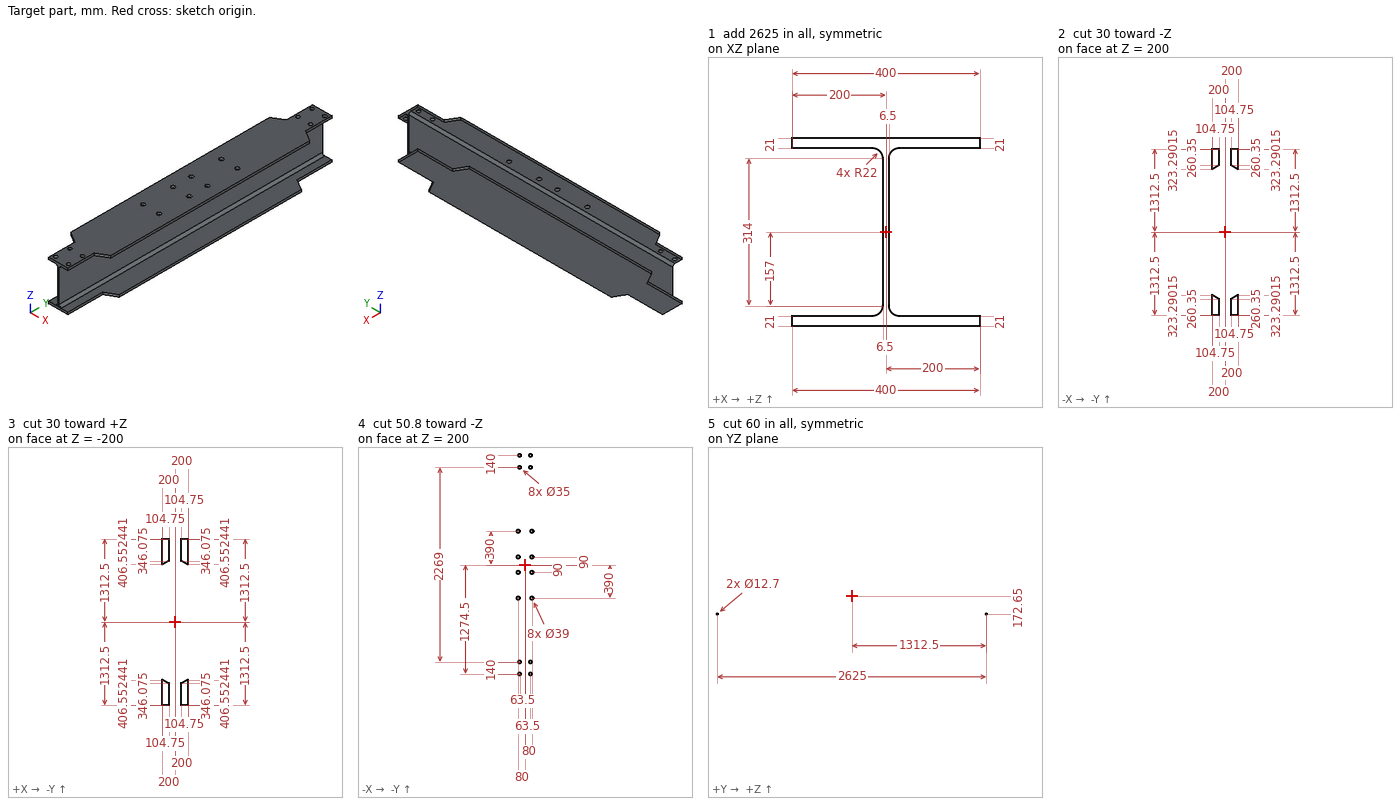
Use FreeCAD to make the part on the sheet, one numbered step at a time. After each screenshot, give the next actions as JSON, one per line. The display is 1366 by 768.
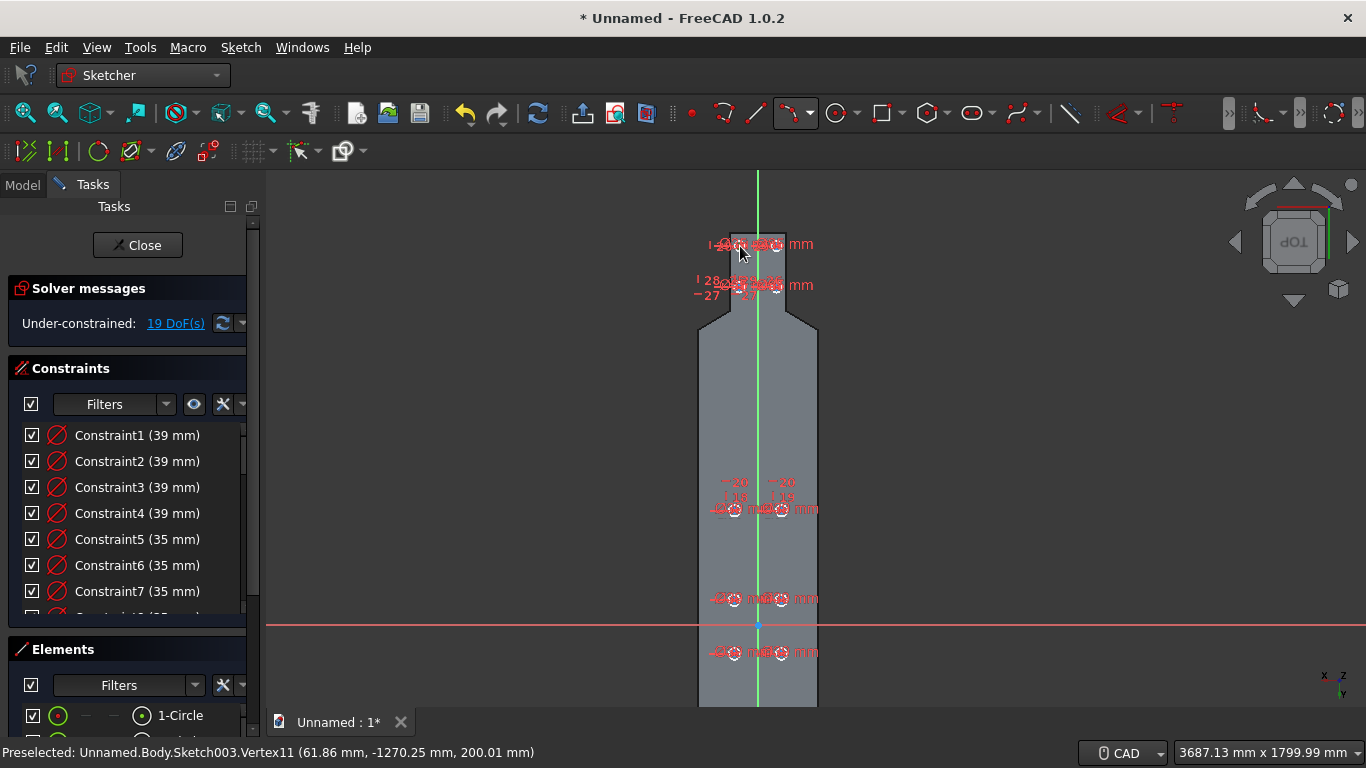
{"action": "left_click", "coordinate": [777, 246]}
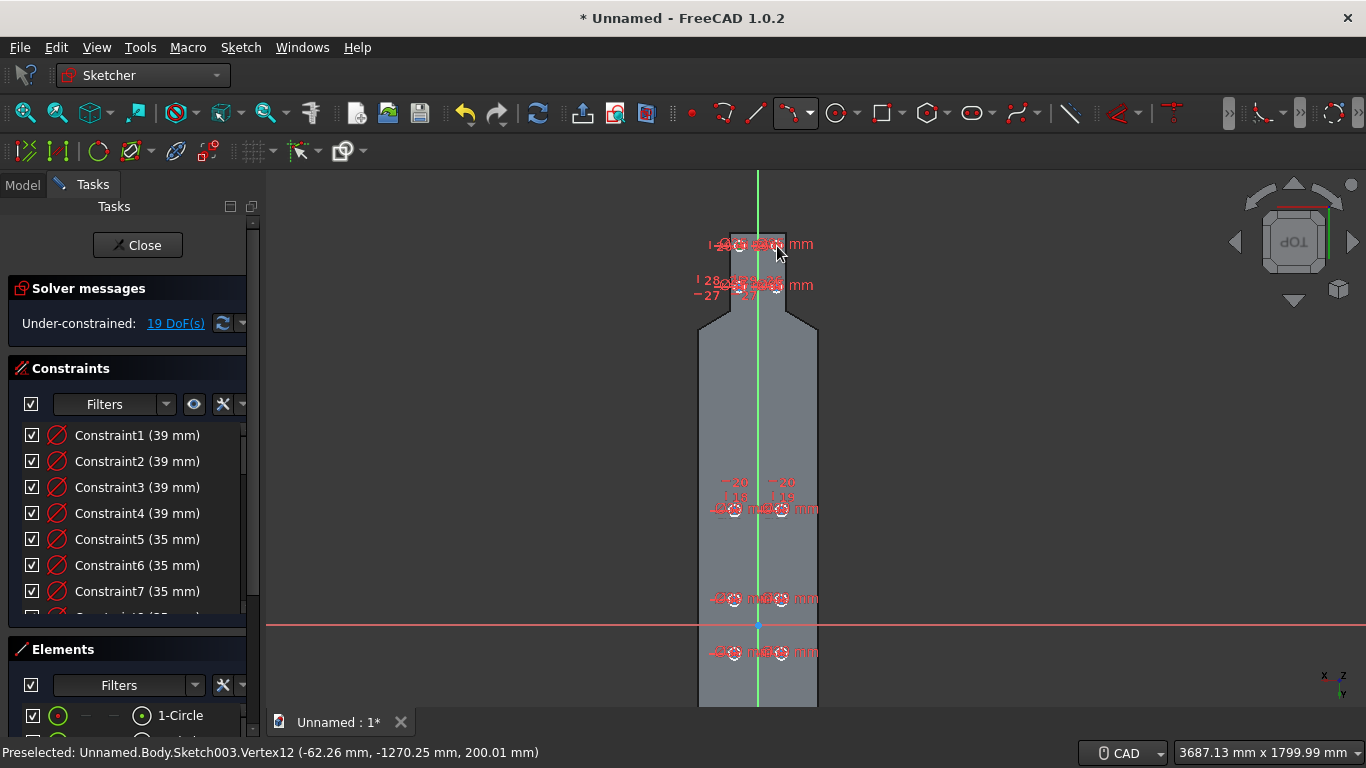
{"action": "key", "text": "h"}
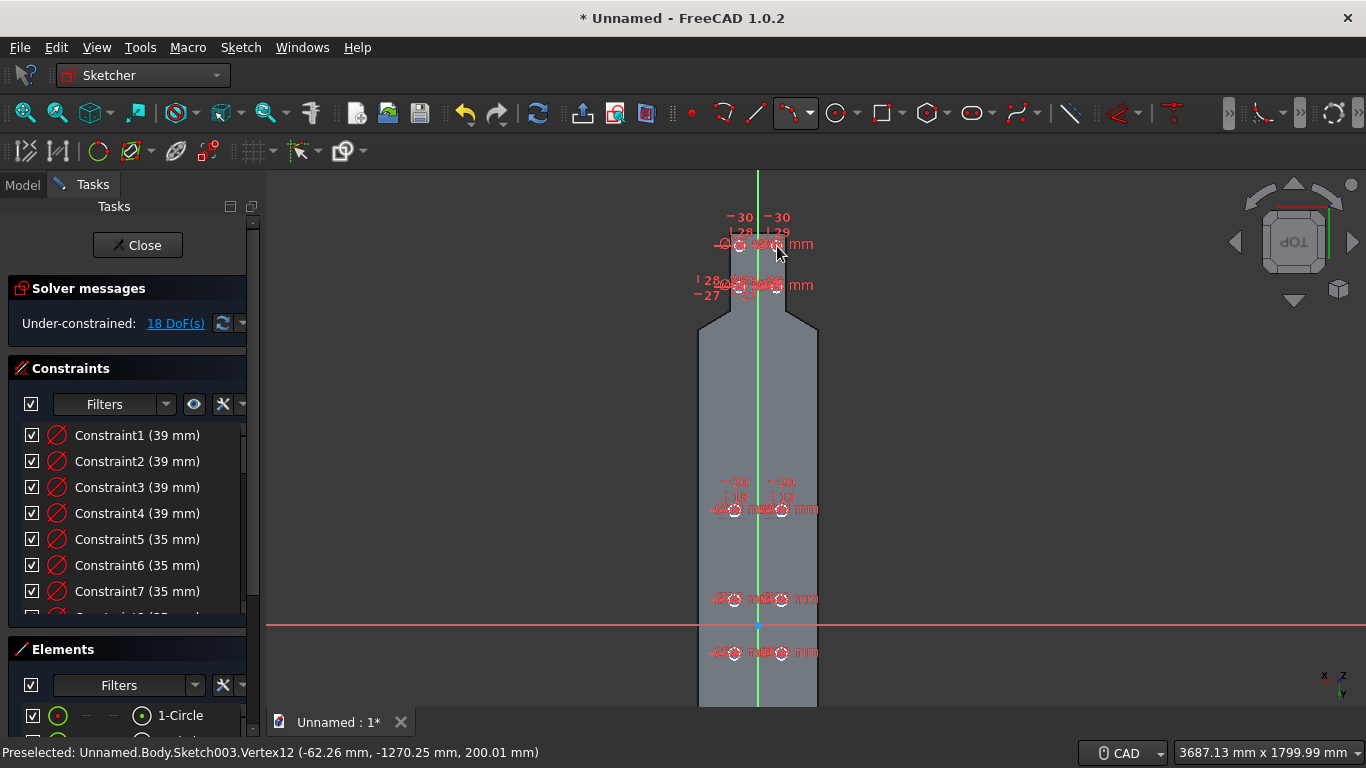
{"action": "scroll", "coordinate": [739, 286], "scroll_direction": "down", "scroll_amount": 4}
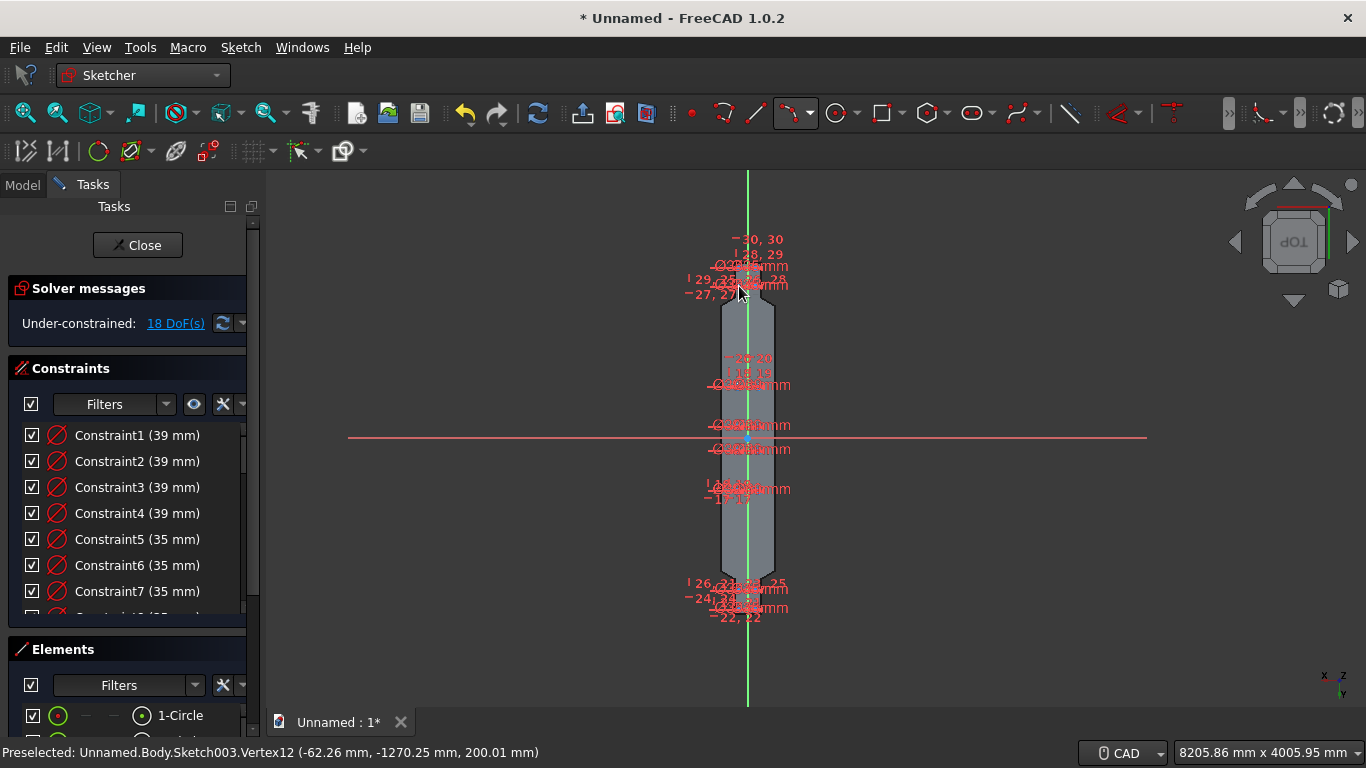
{"action": "left_click", "coordinate": [758, 491]}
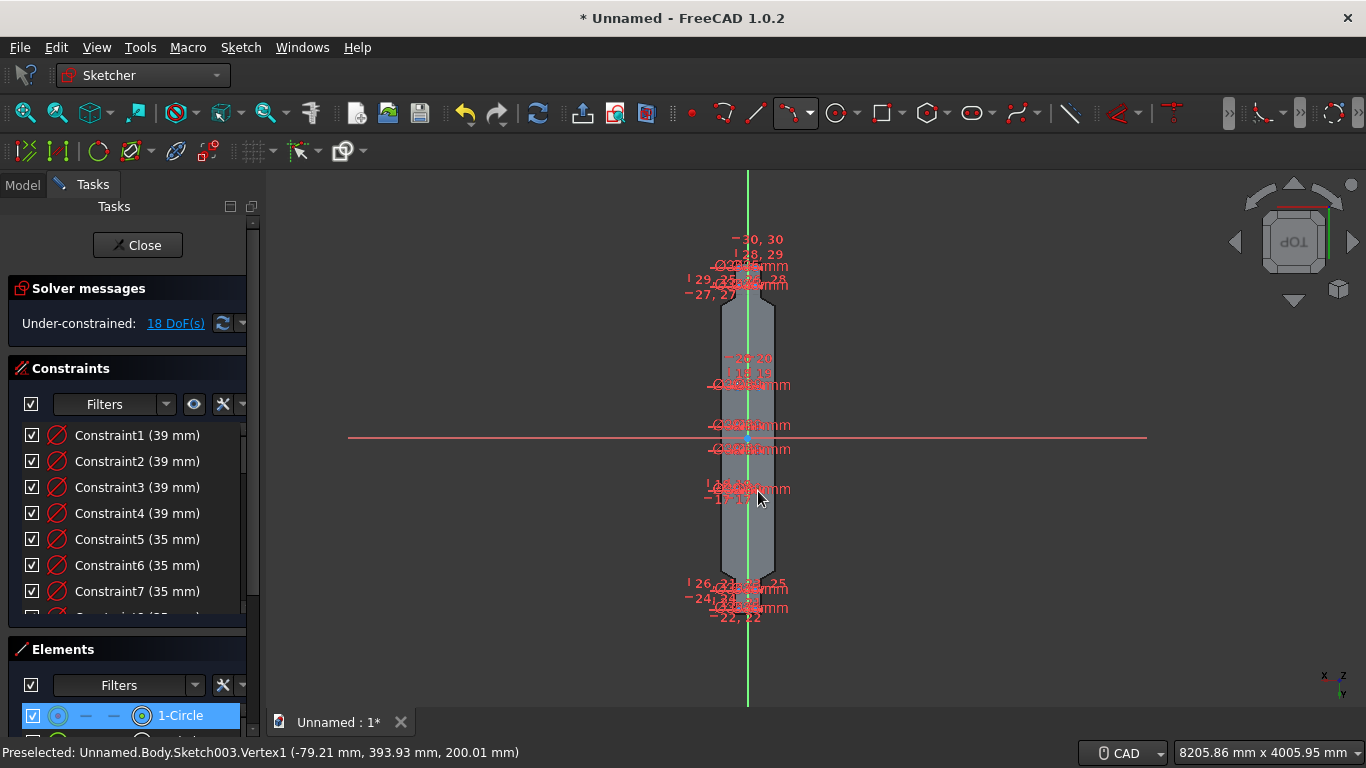
{"action": "left_click", "coordinate": [758, 451]}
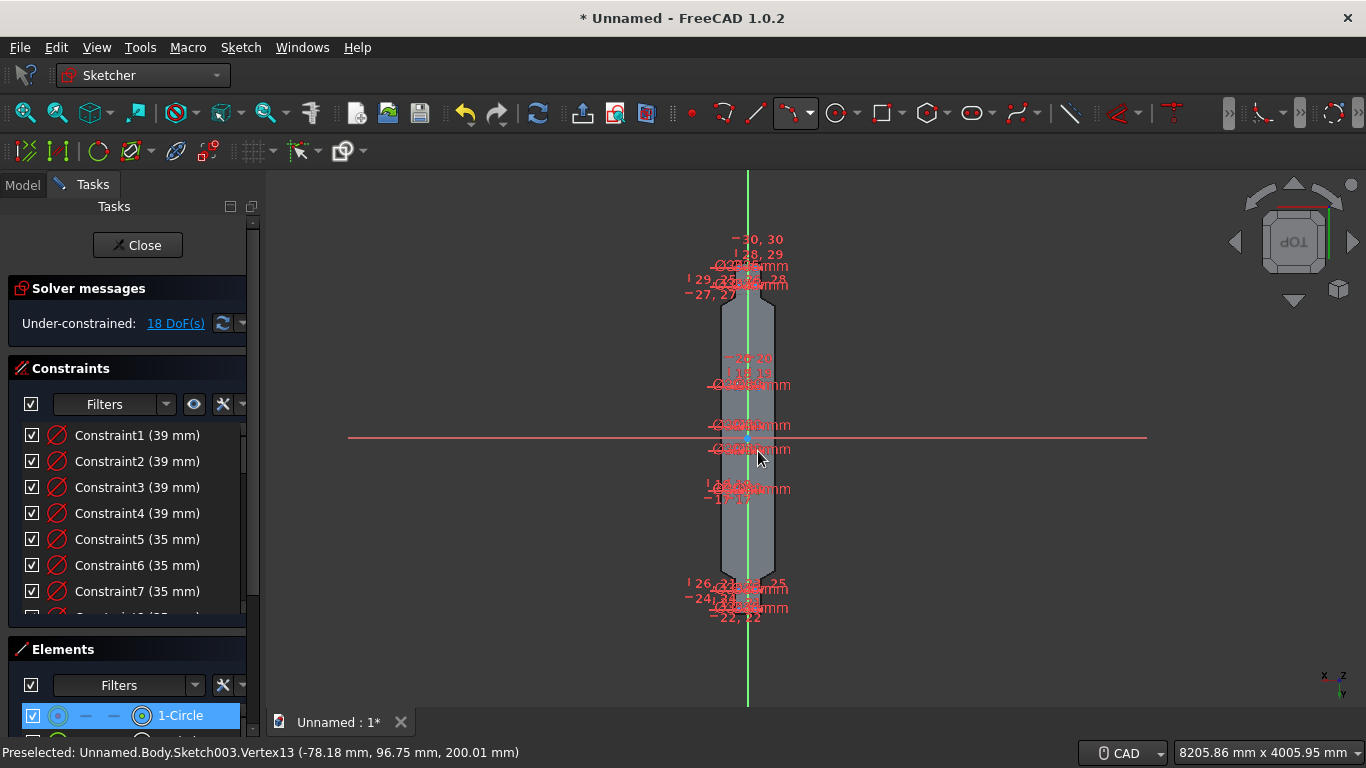
{"action": "key", "text": "v"}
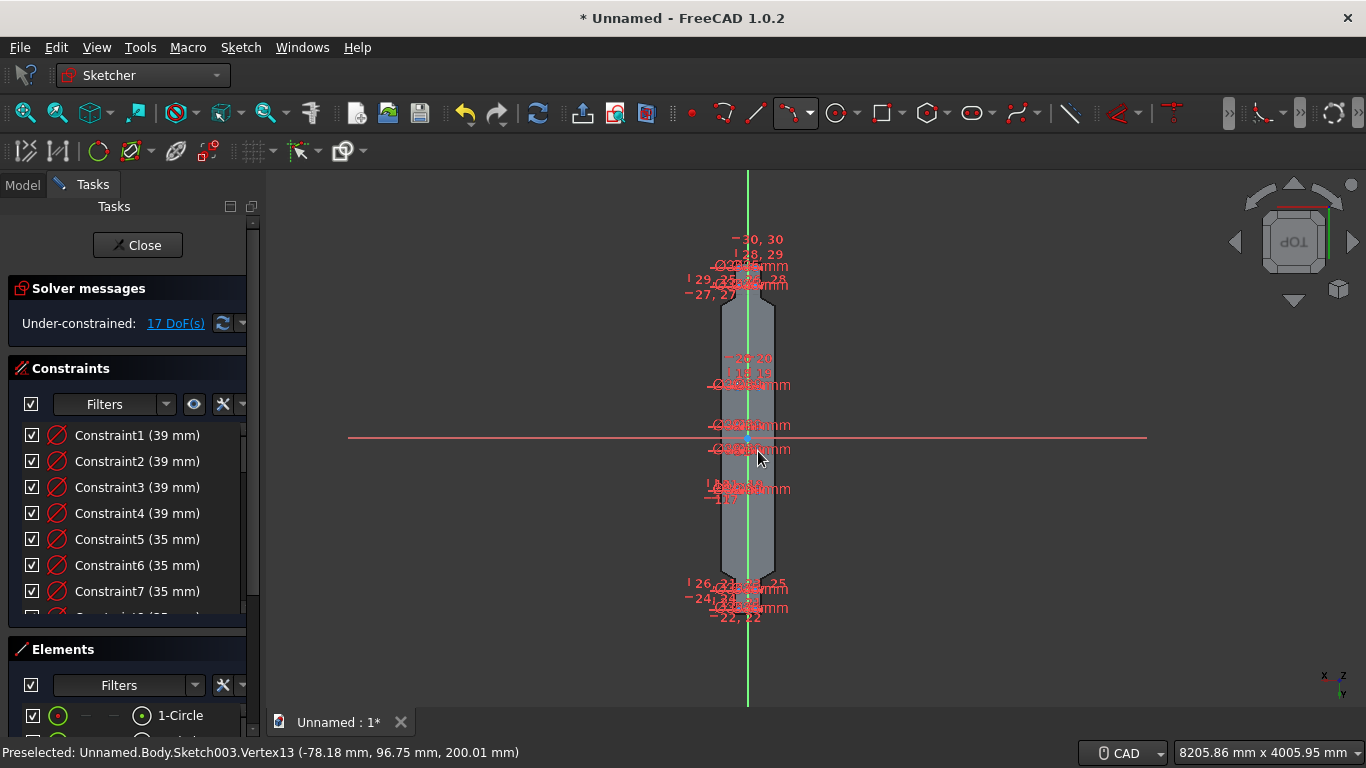
{"action": "left_click", "coordinate": [737, 491]}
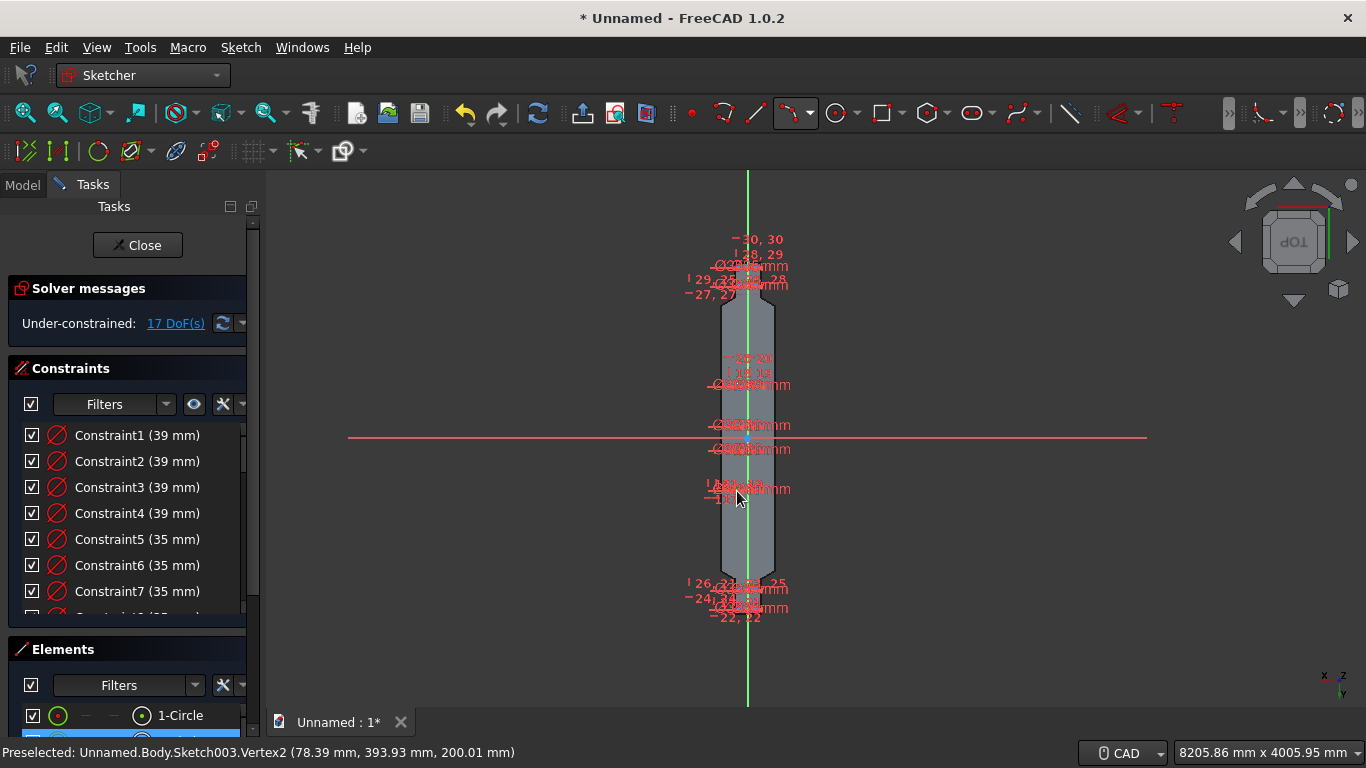
{"action": "scroll", "coordinate": [737, 451], "scroll_direction": "up", "scroll_amount": 4}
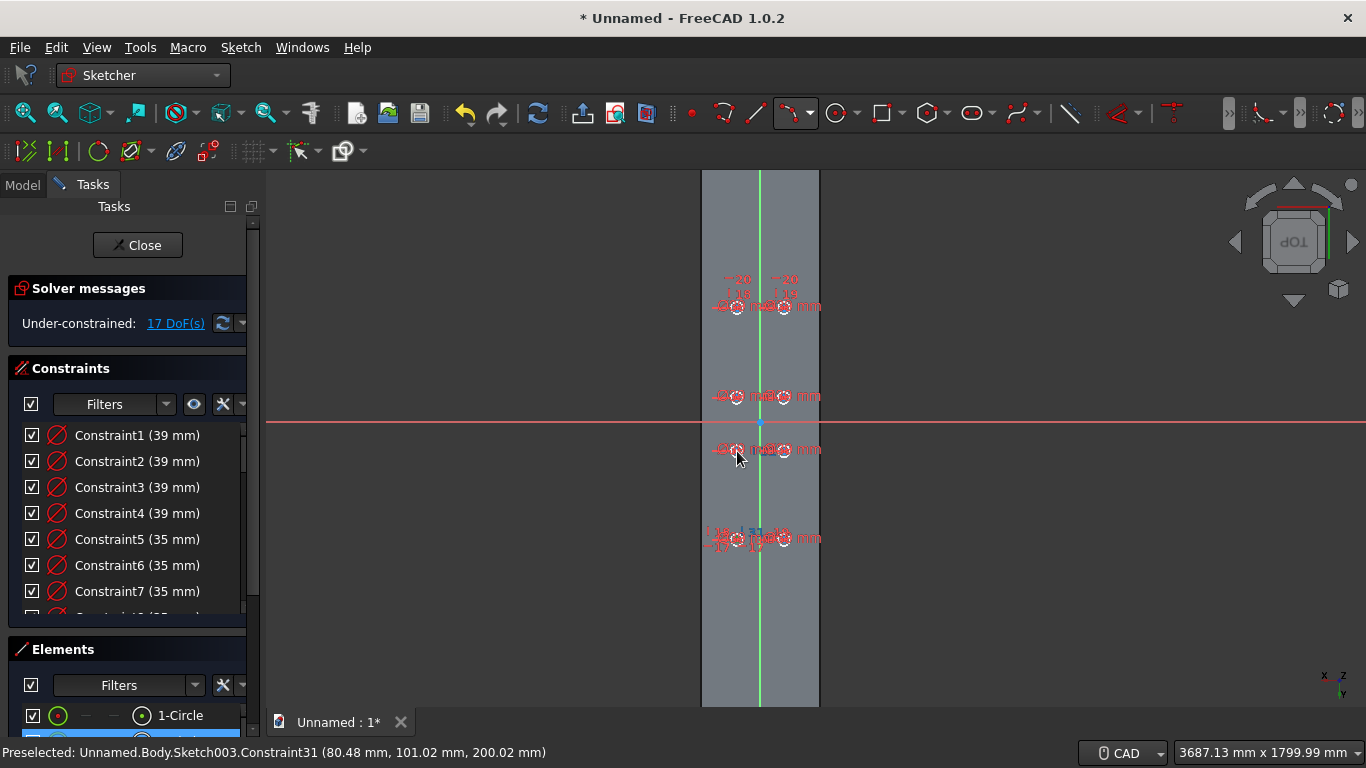
{"action": "left_click", "coordinate": [737, 451]}